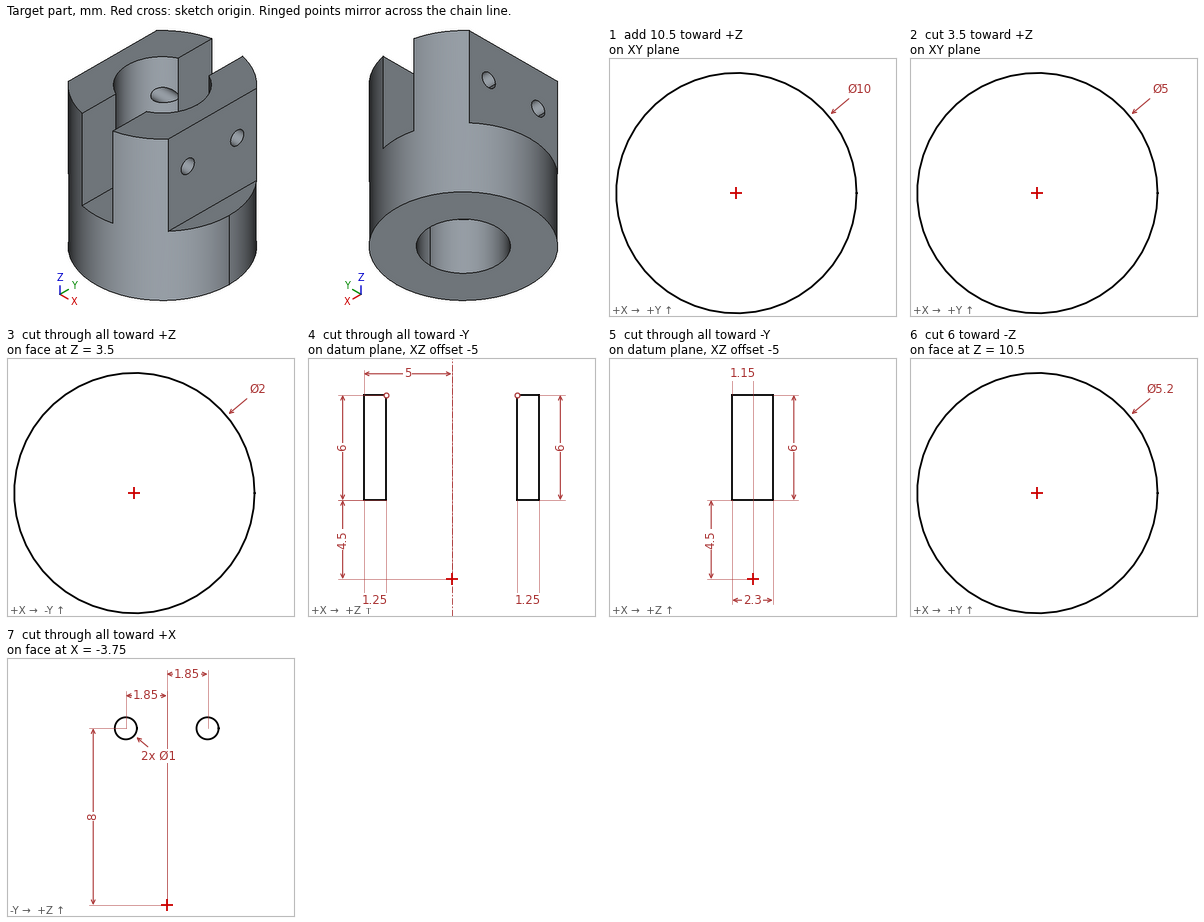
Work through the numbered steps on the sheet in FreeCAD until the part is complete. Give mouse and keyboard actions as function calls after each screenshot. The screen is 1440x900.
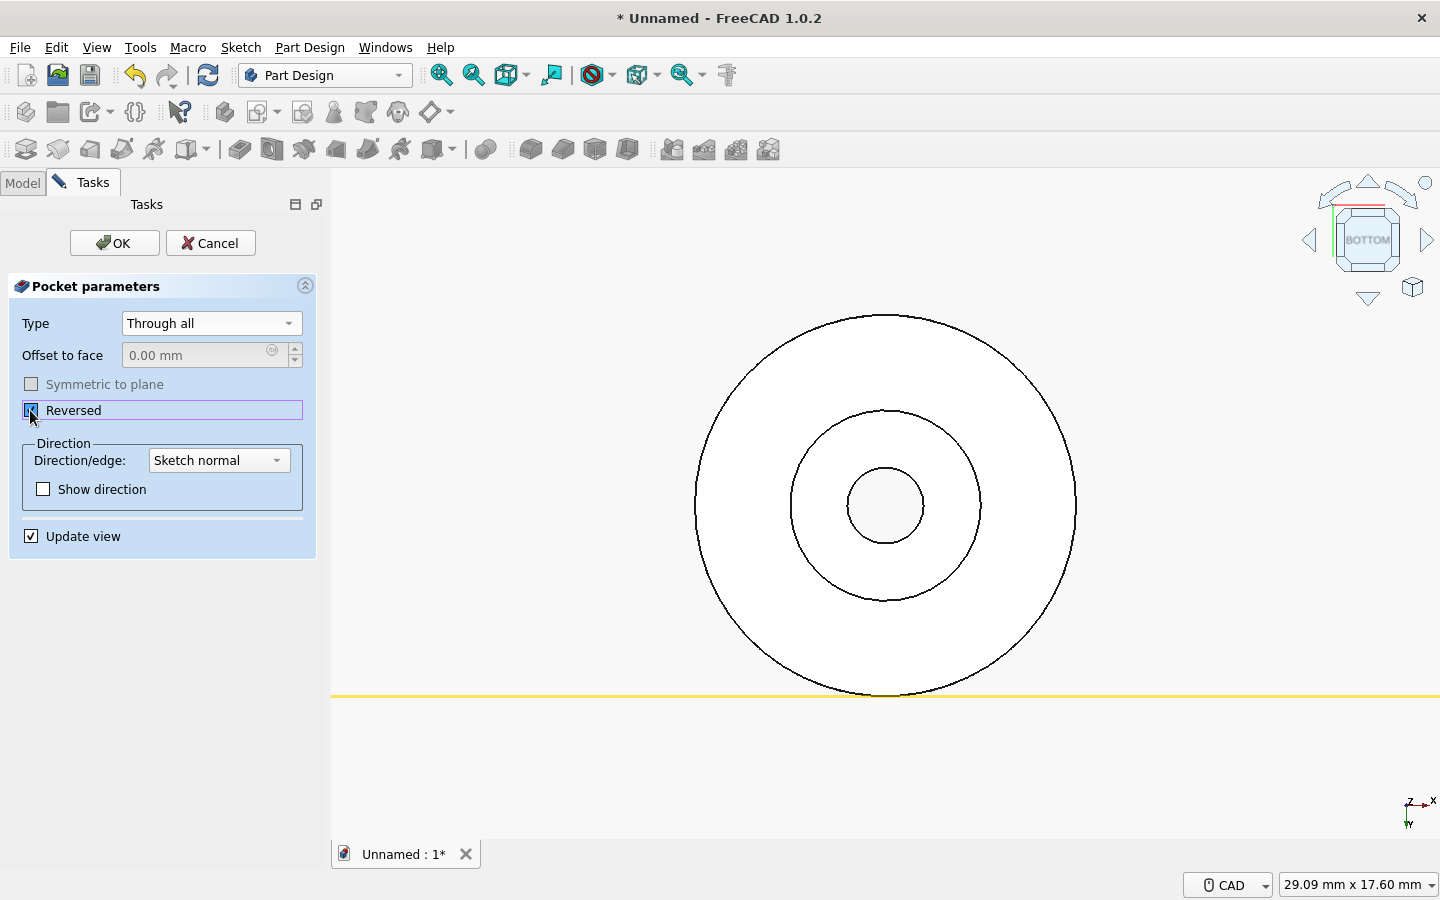
click(115, 243)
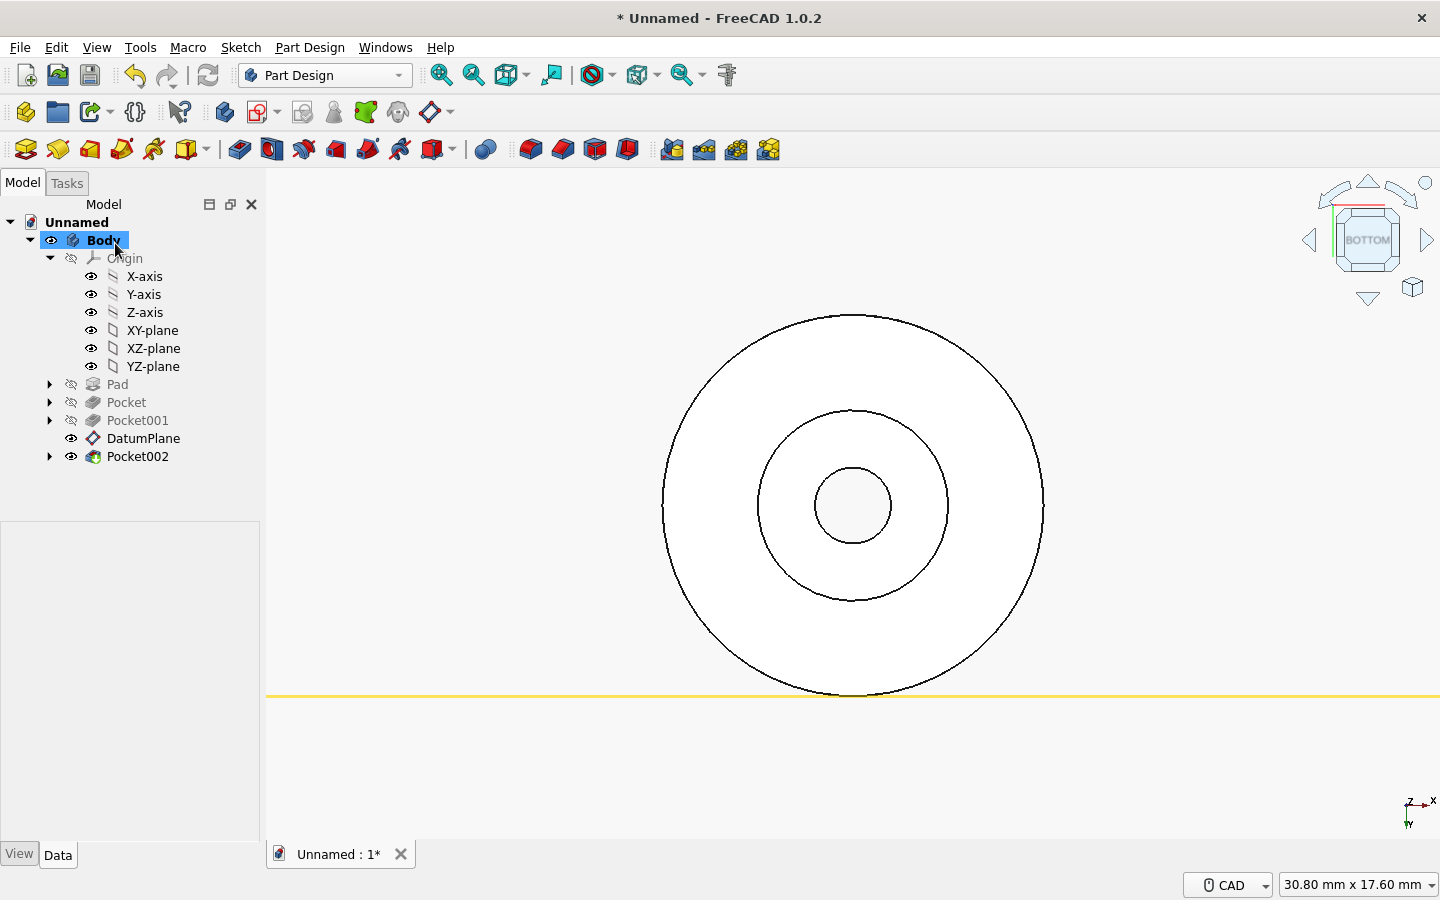
click(116, 438)
key(space)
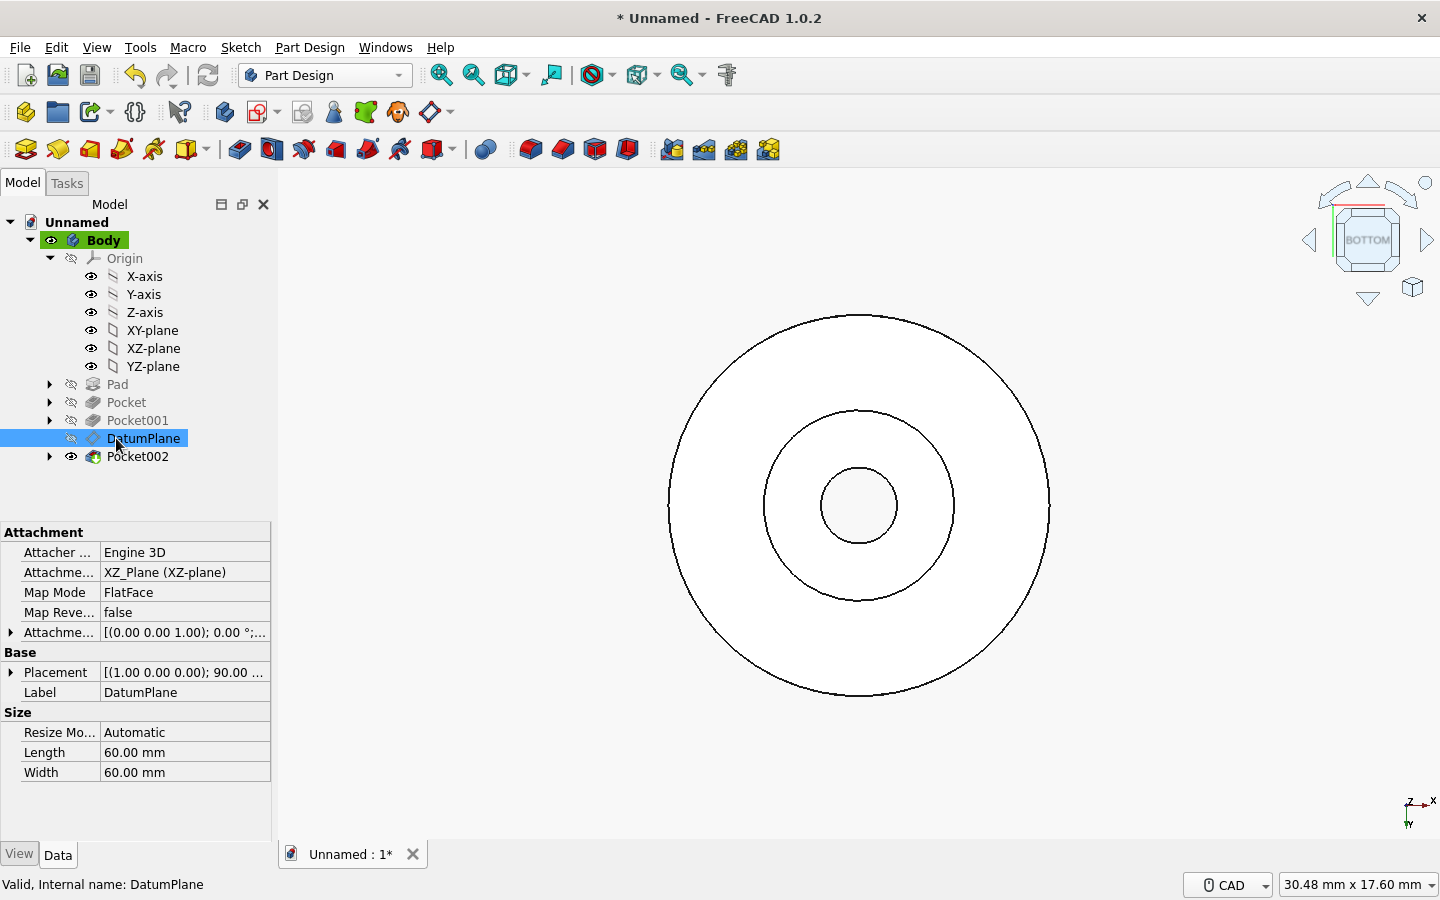
click(136, 348)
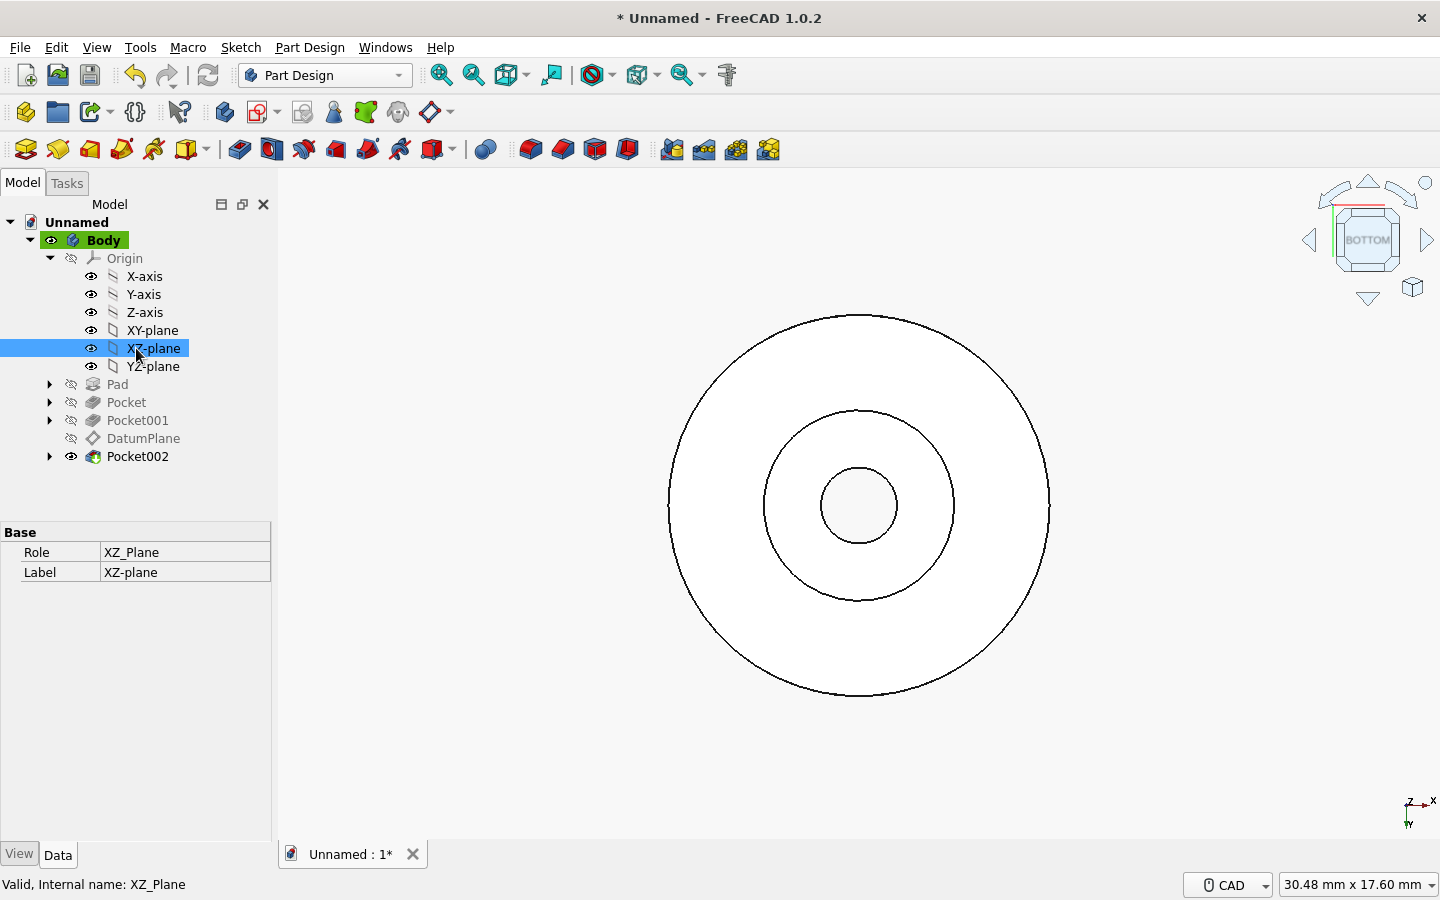
click(430, 112)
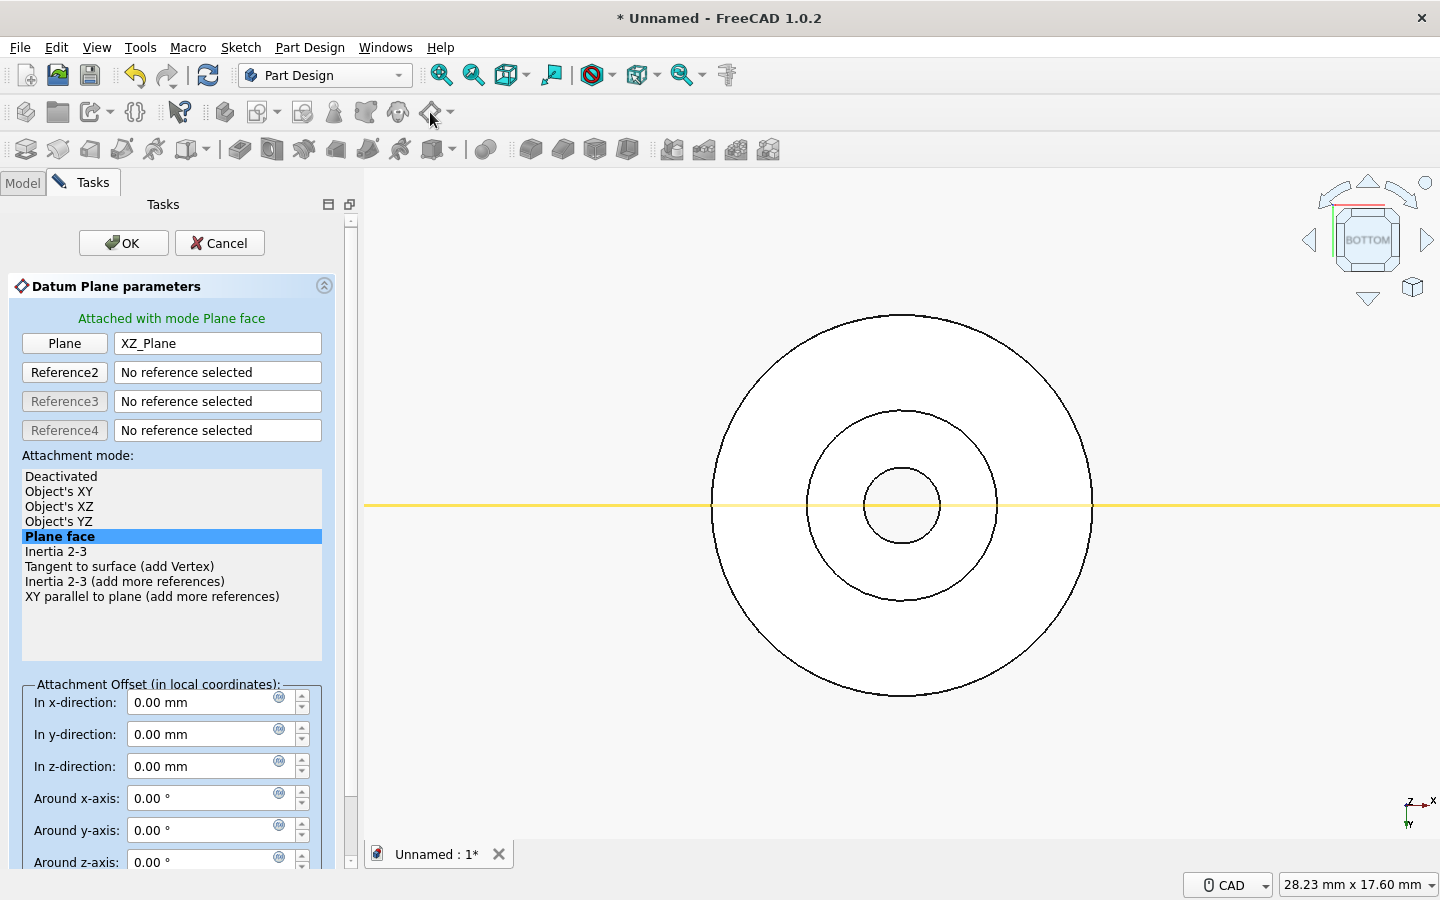
triple_click(210, 766)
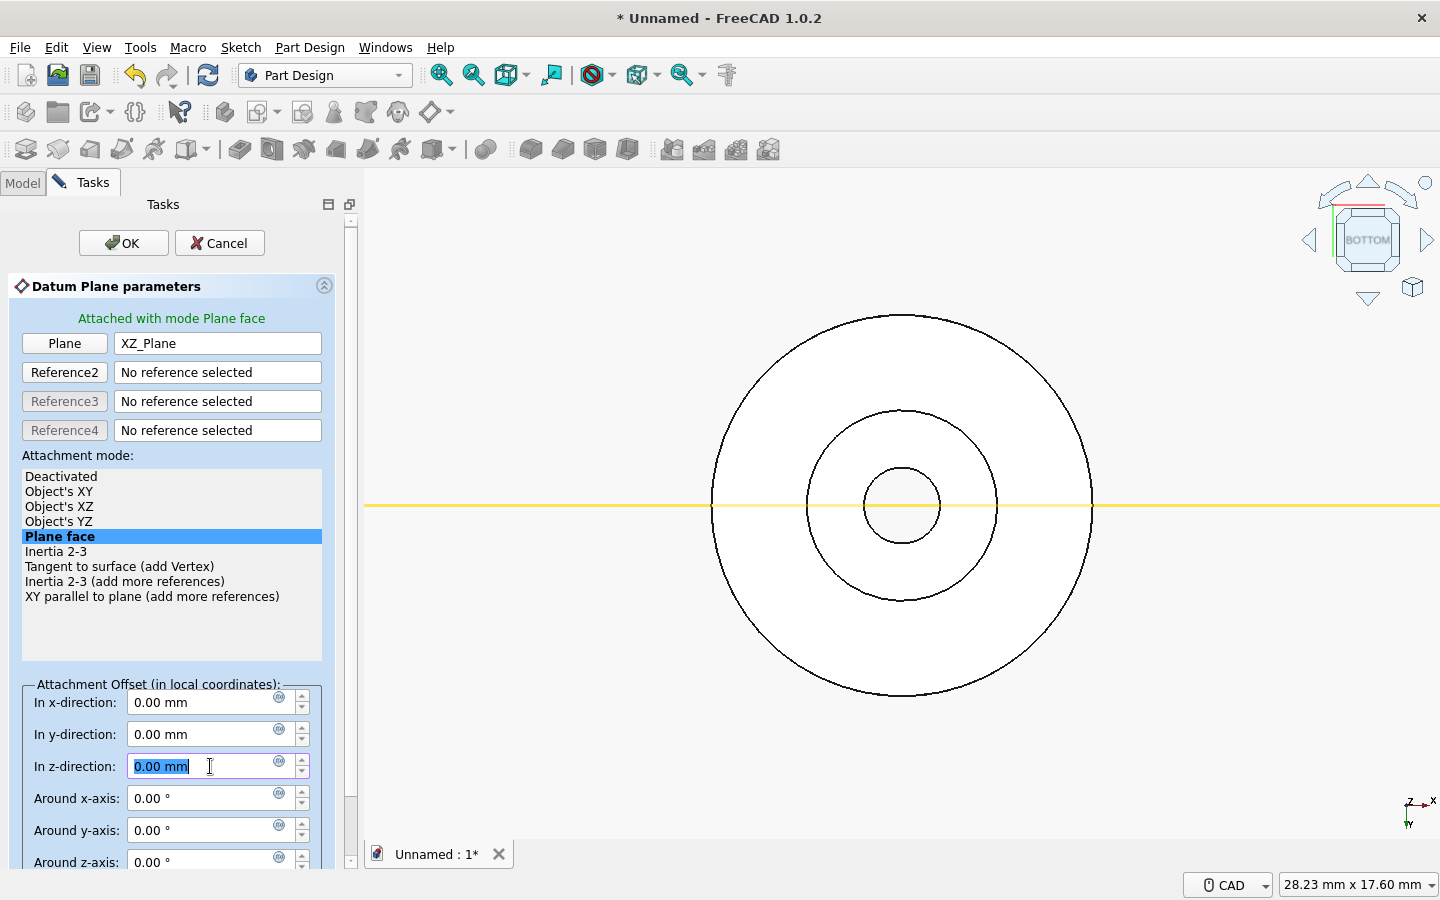
text(-5)
key(Tab)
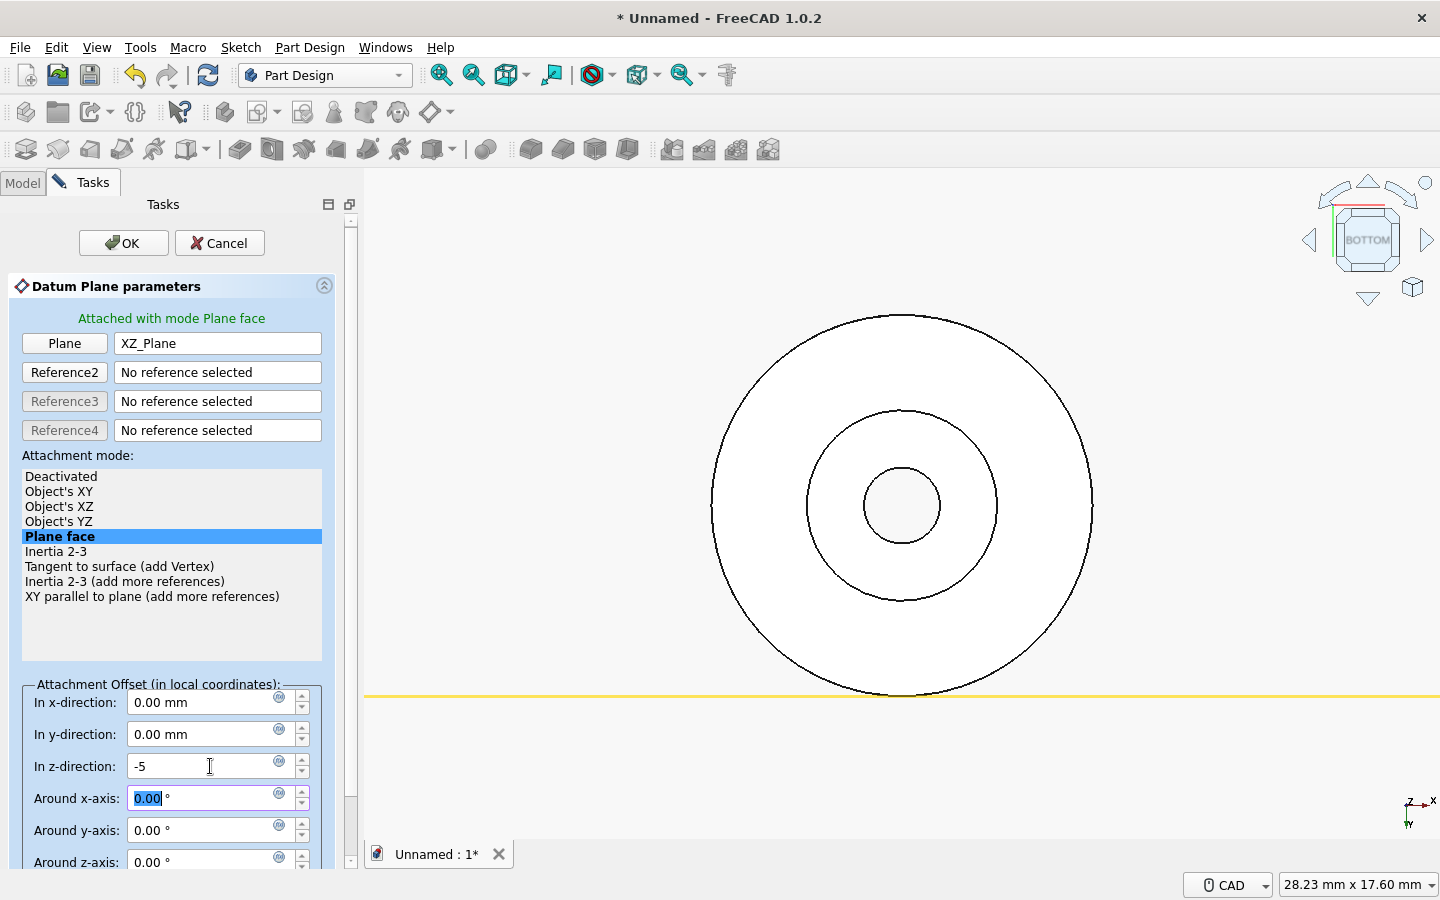
click(124, 243)